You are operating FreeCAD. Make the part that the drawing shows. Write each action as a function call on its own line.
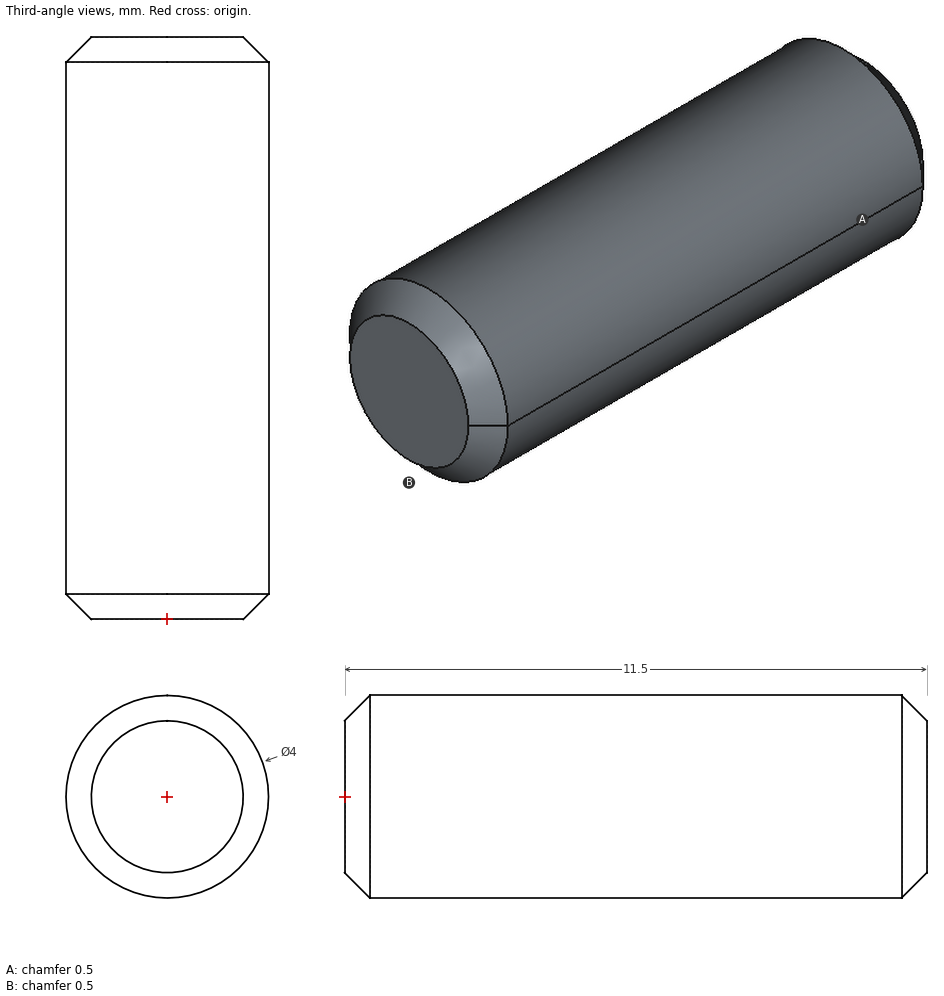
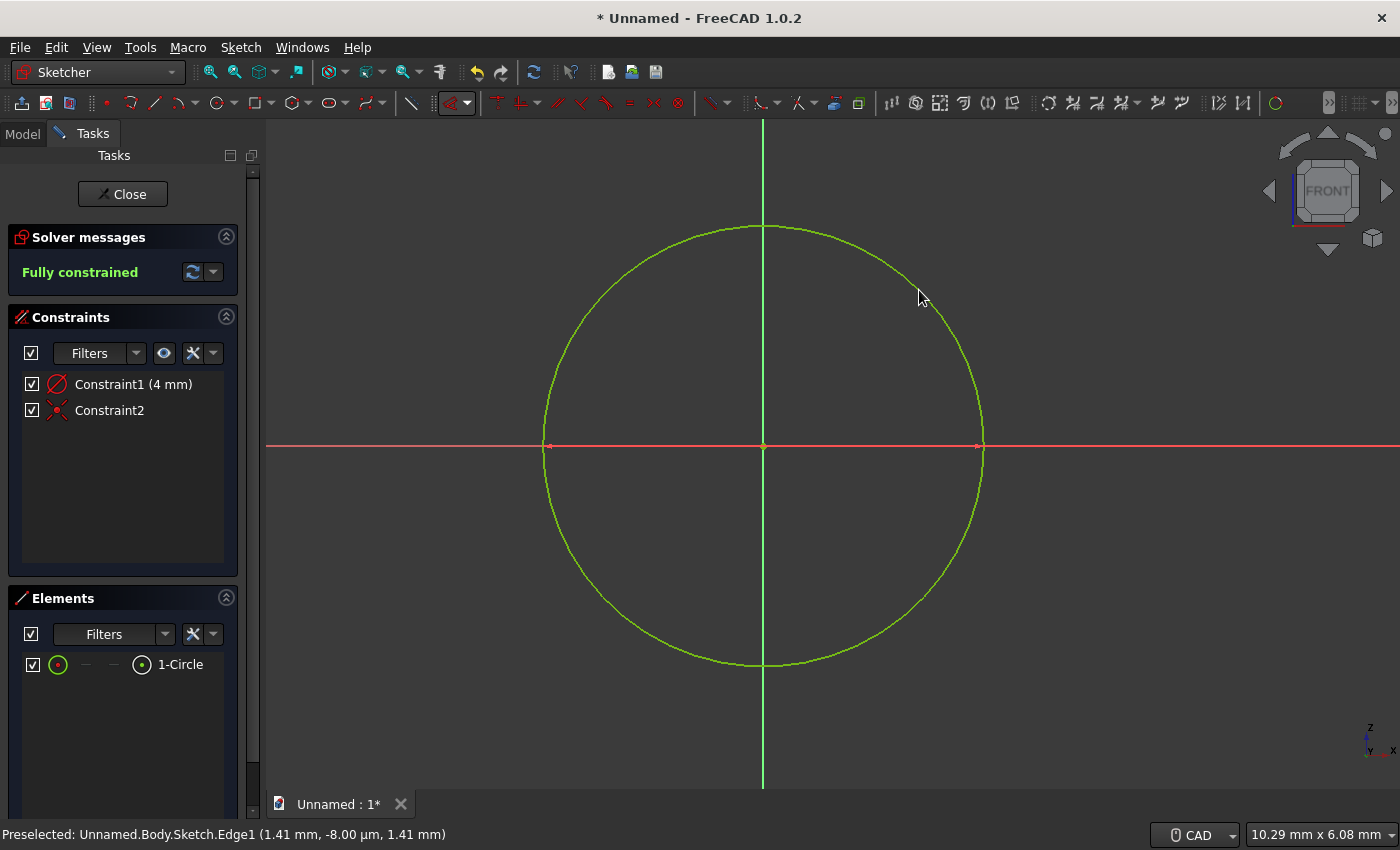
click(123, 194)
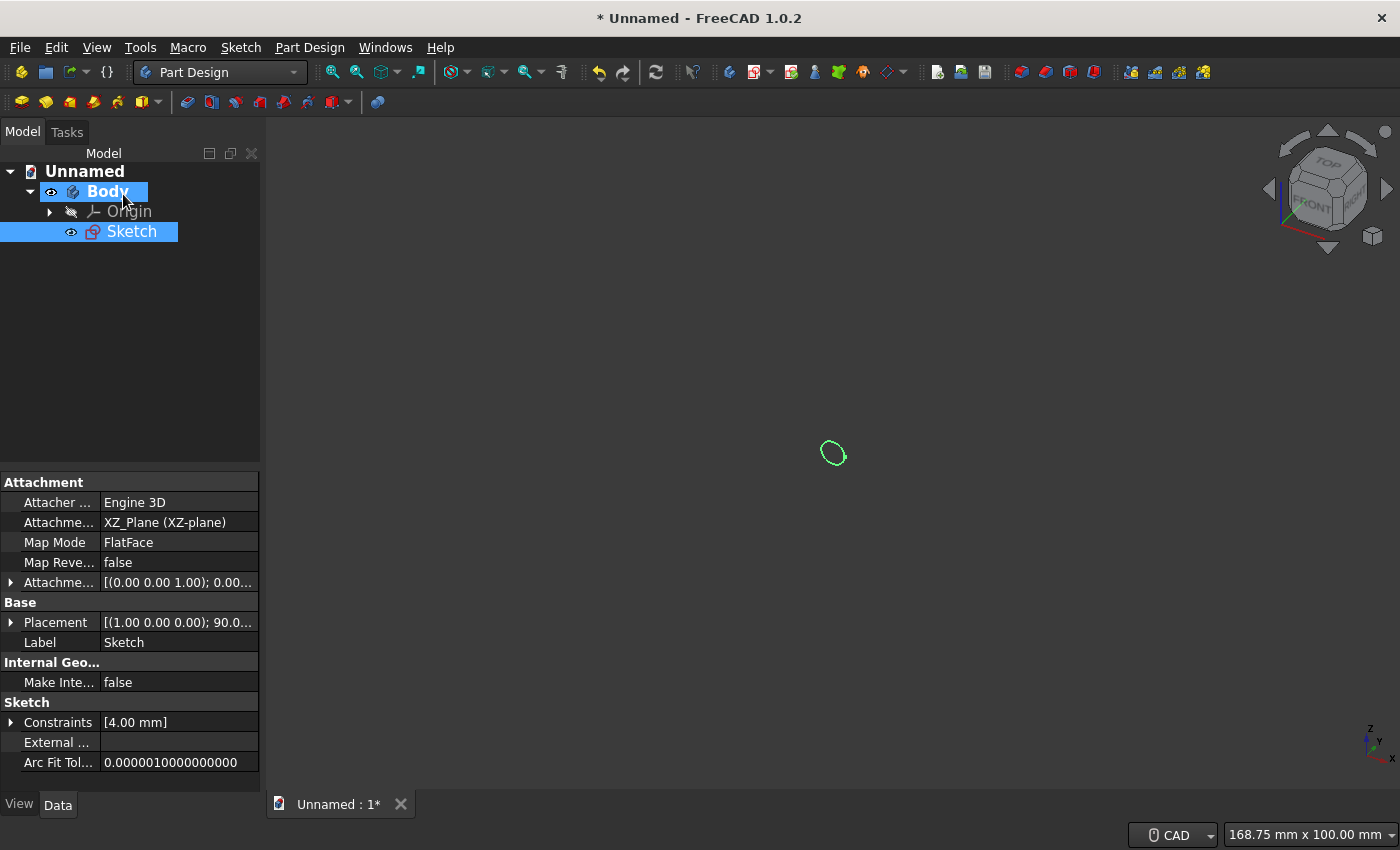
click(22, 102)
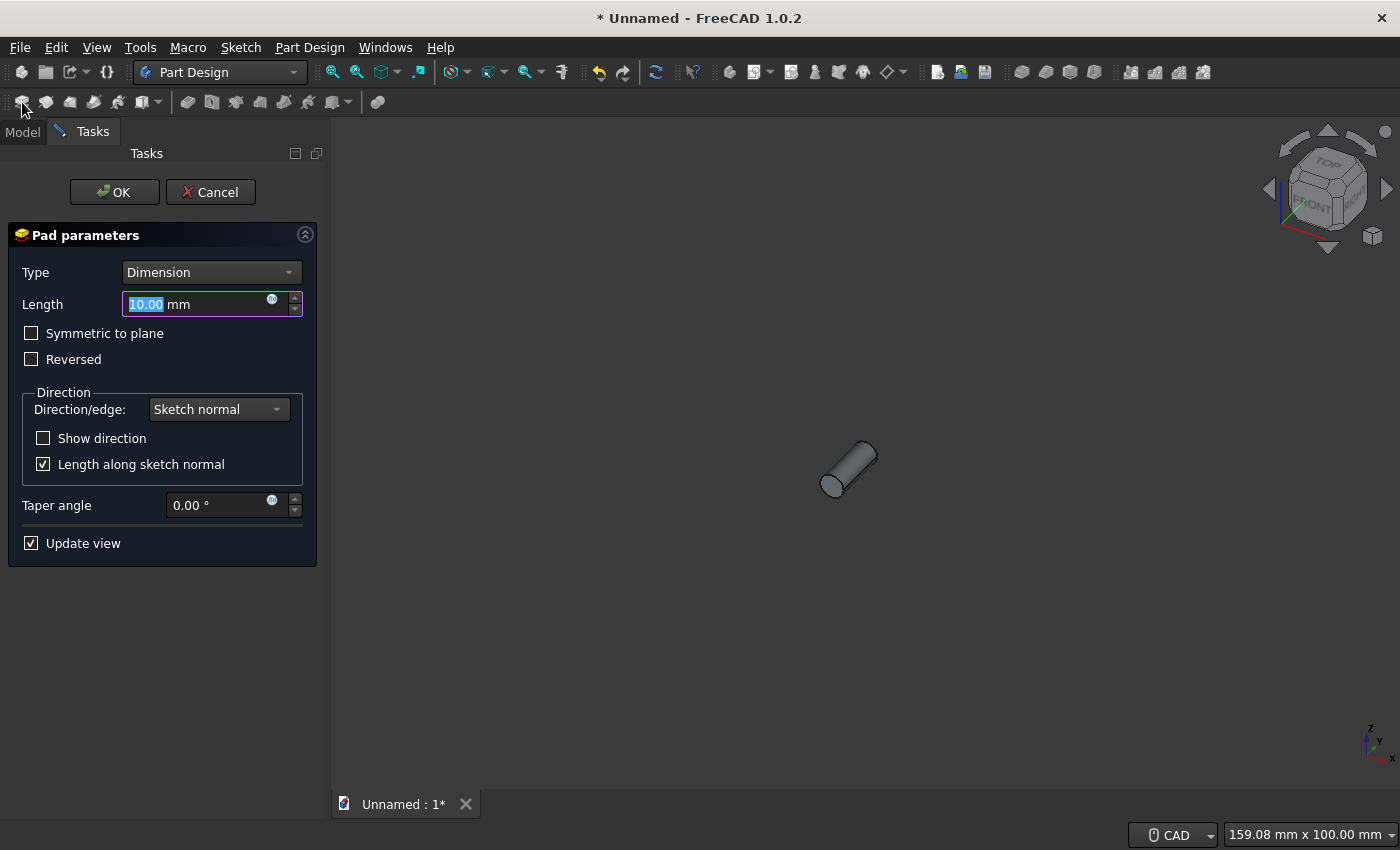
text(11.5)
key(Tab)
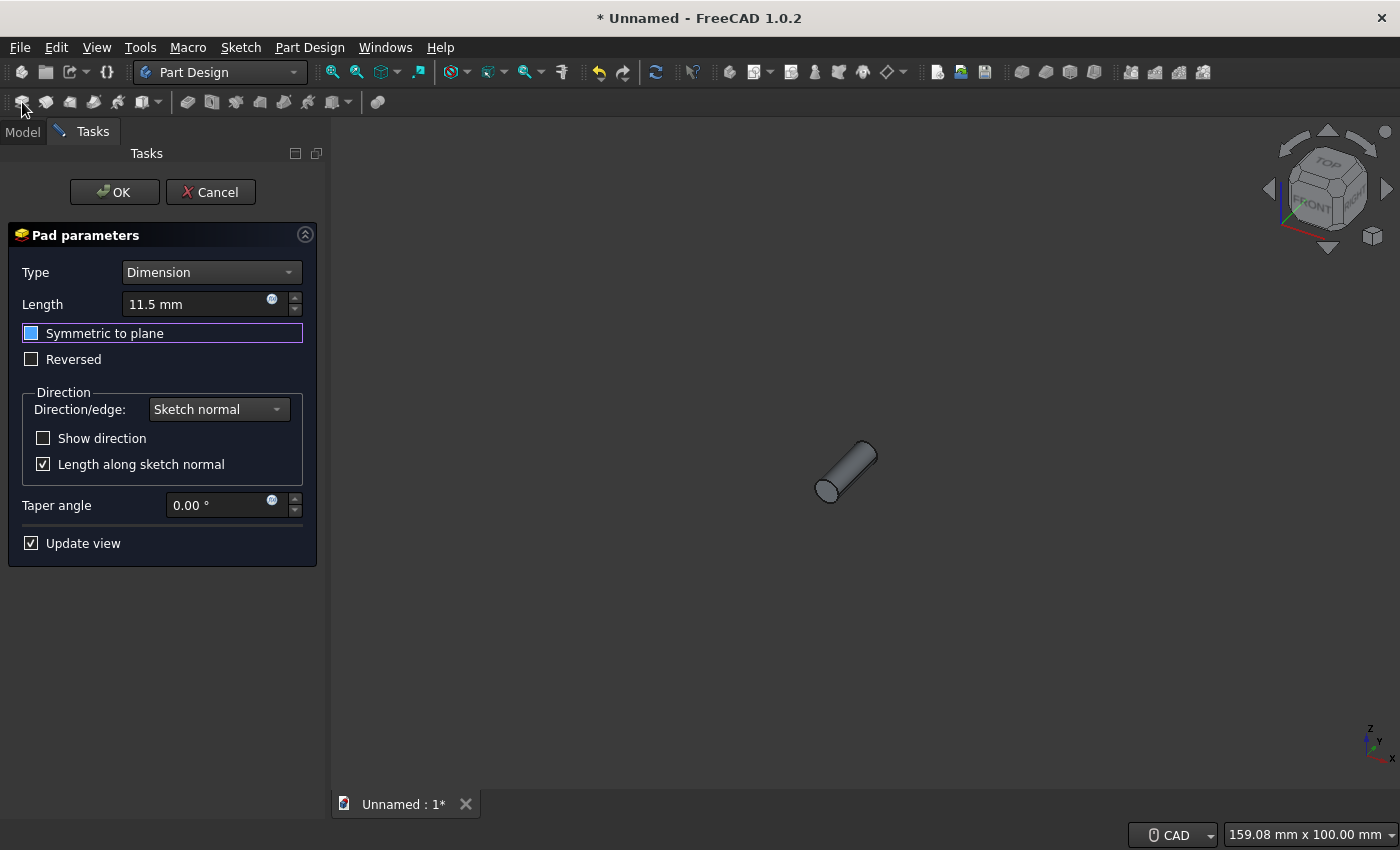
click(30, 359)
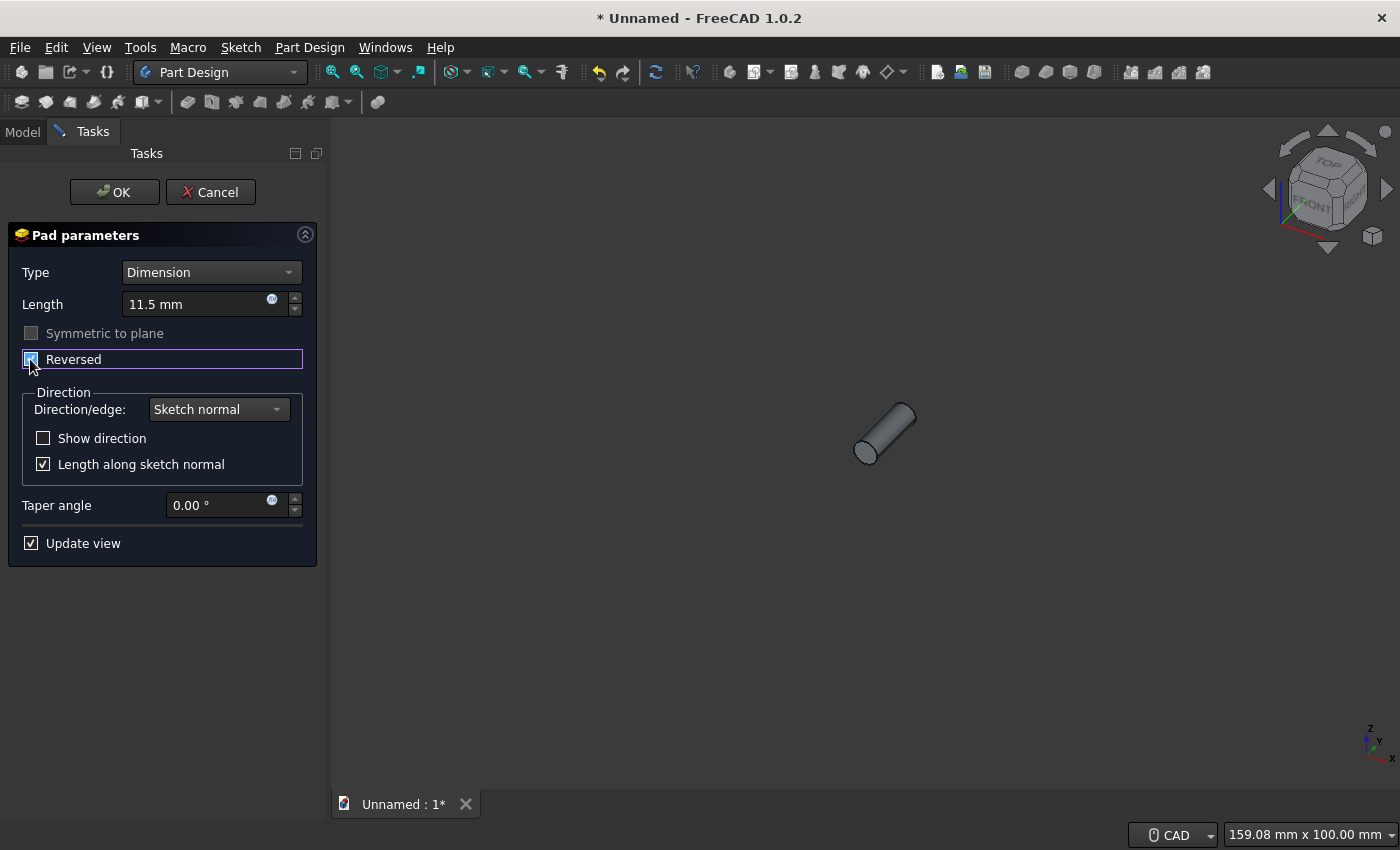
click(115, 192)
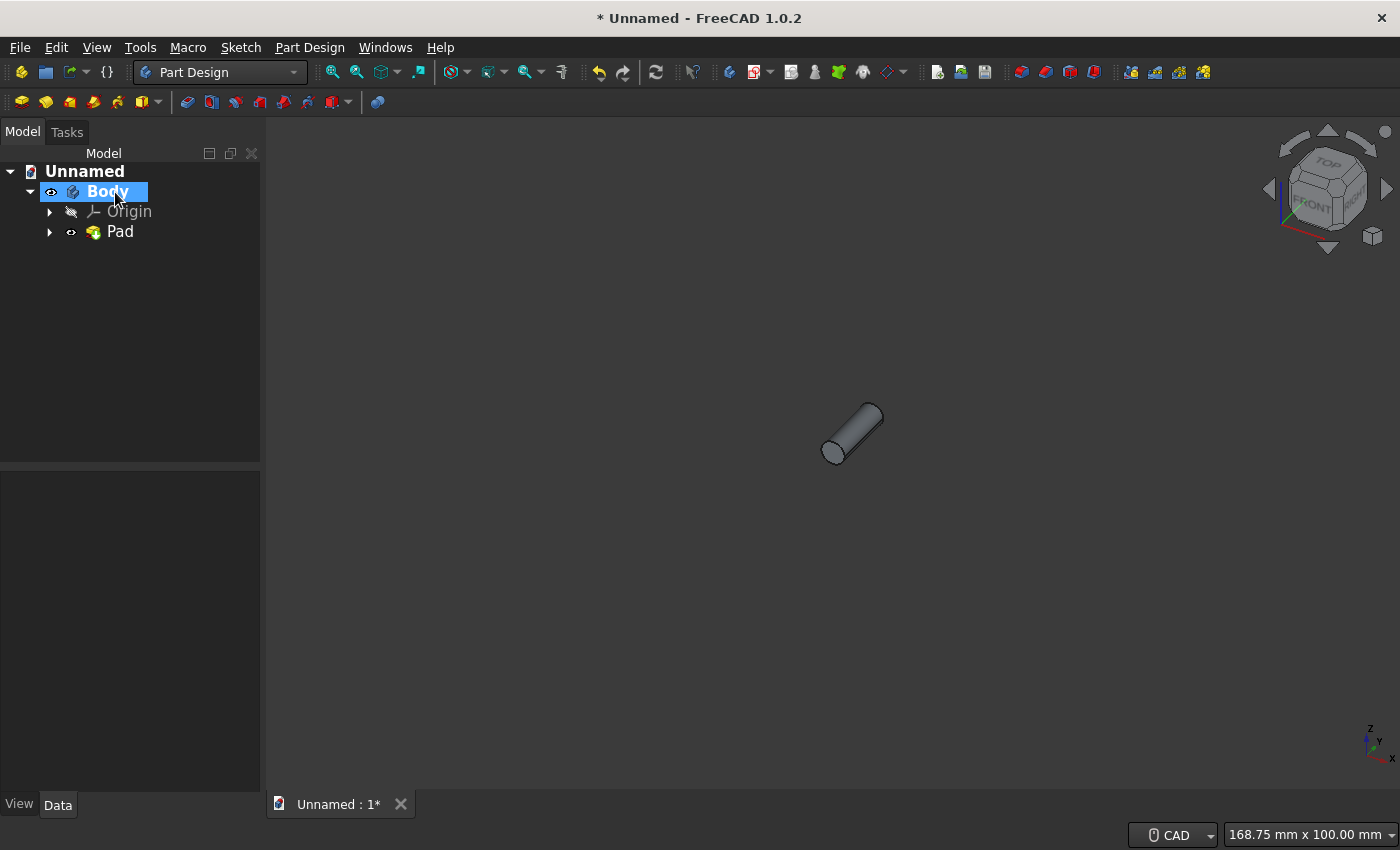
click(334, 72)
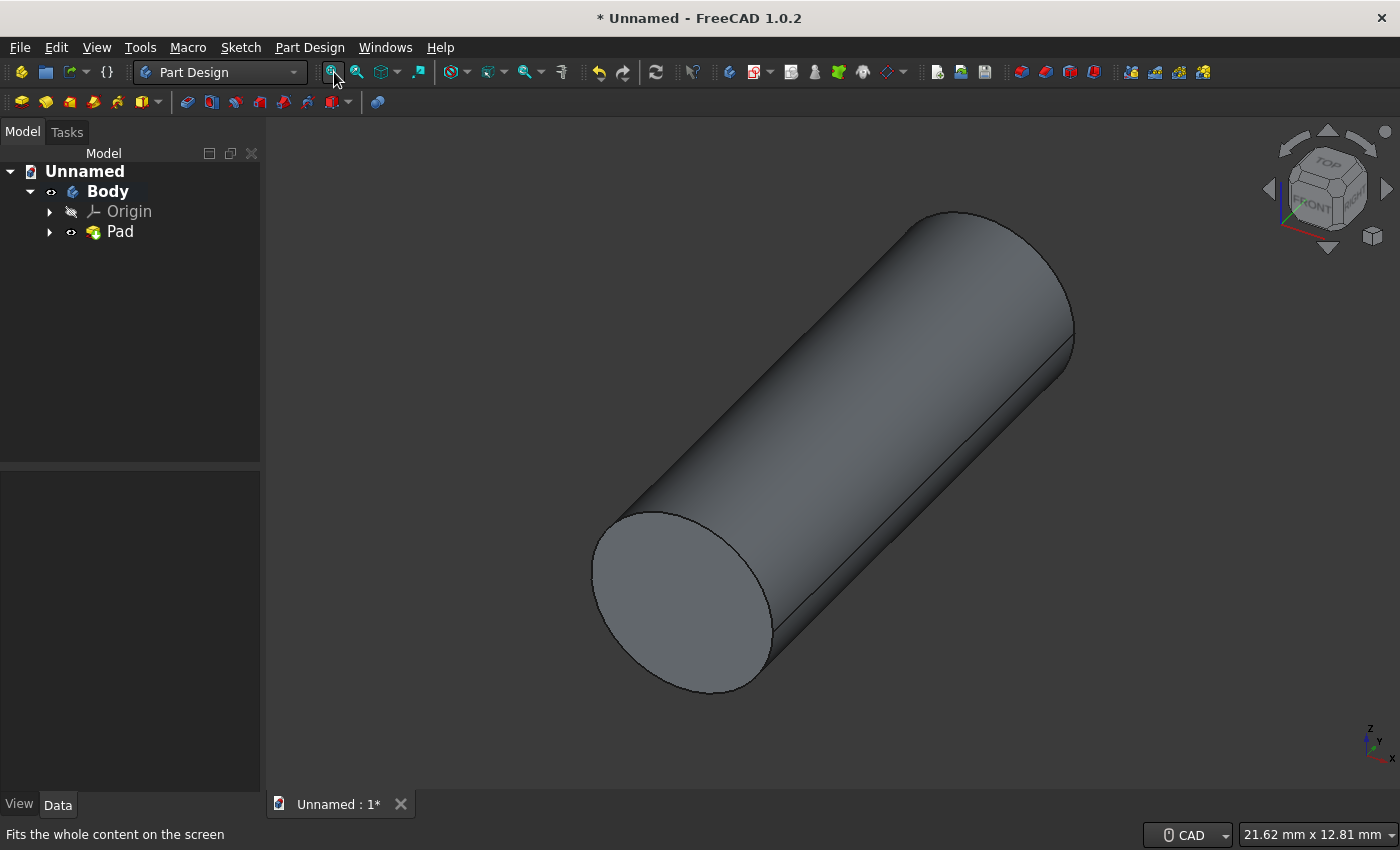
key(0)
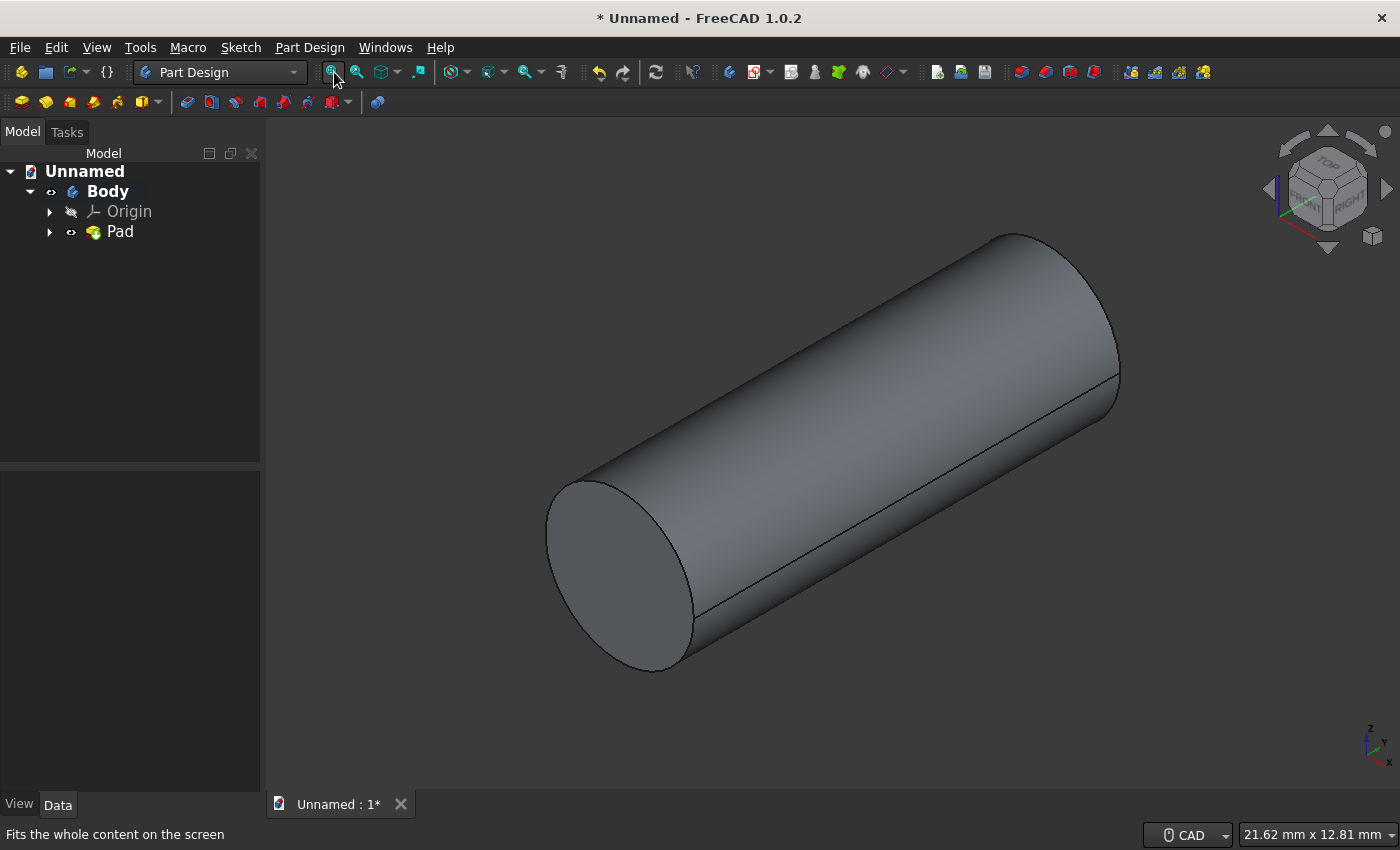
key(2)